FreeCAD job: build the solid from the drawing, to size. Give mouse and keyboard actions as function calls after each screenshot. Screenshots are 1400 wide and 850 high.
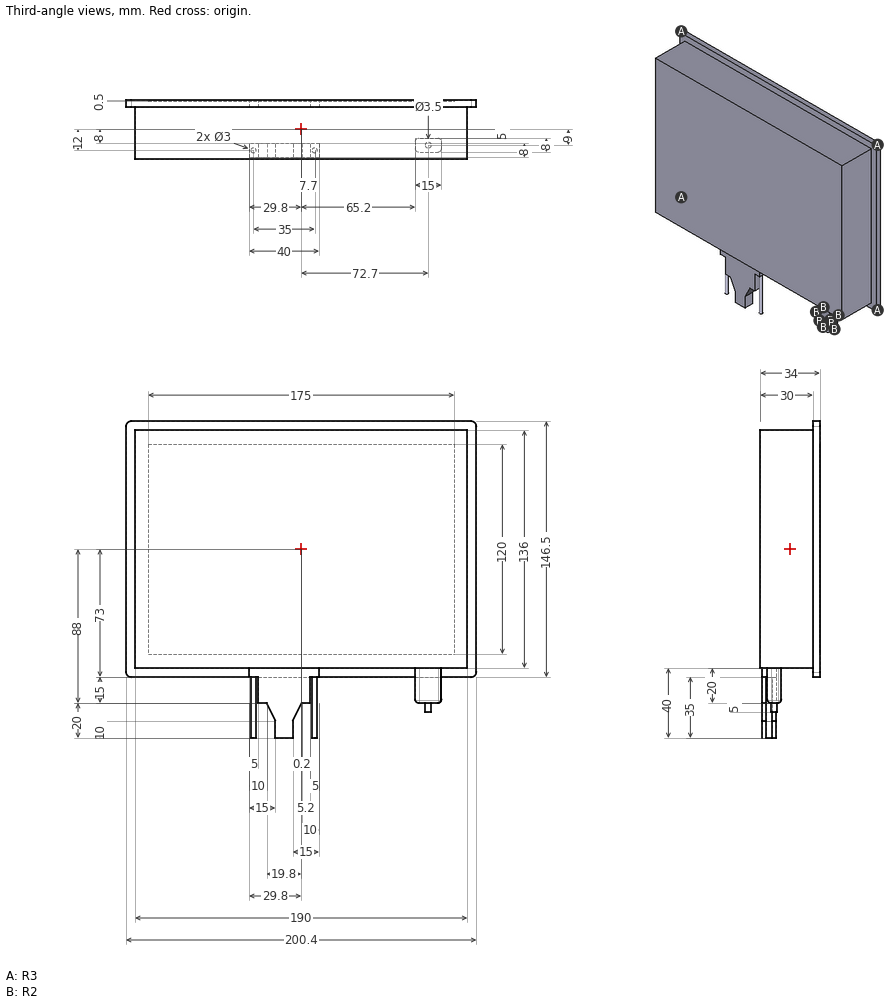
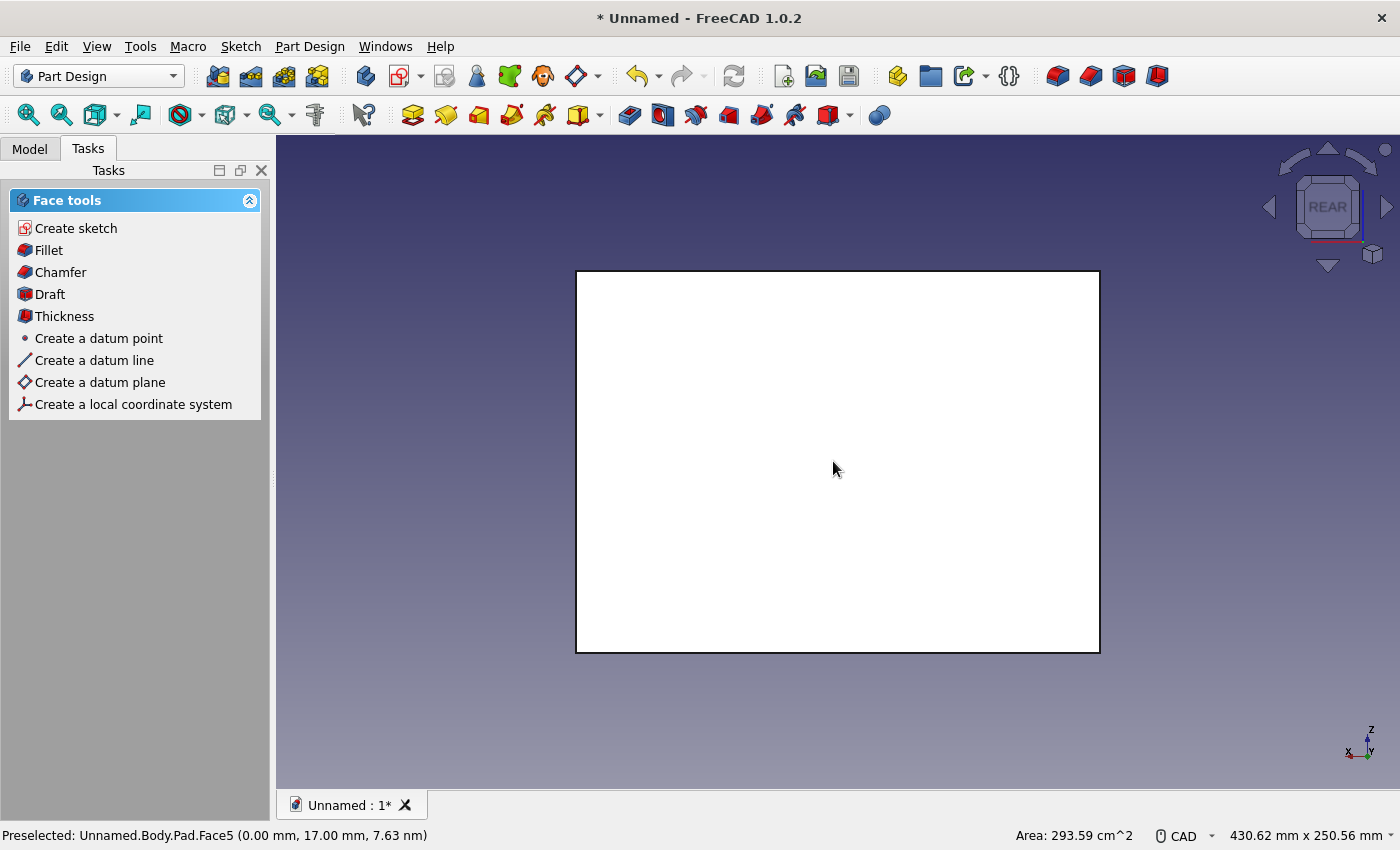
click(398, 76)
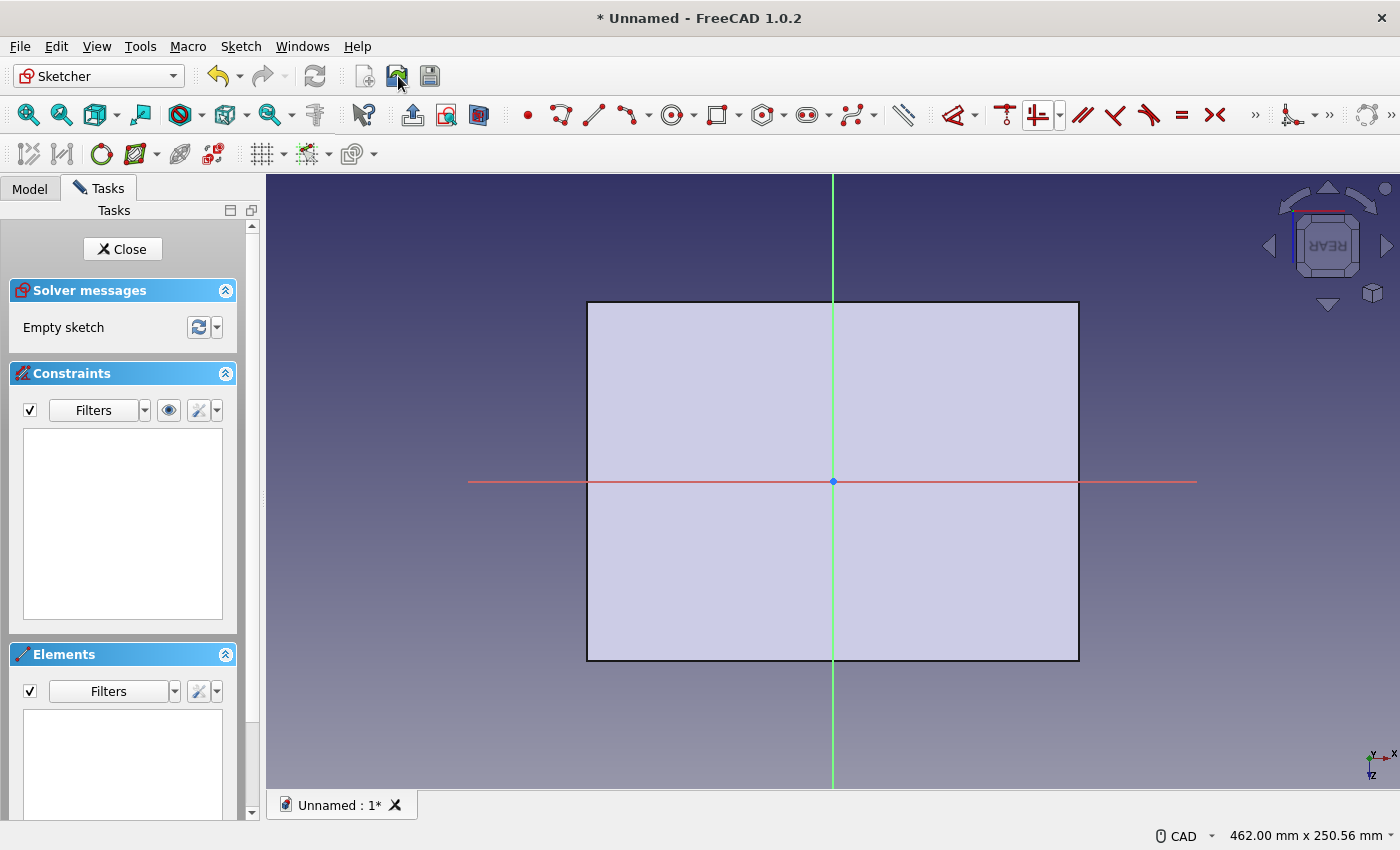
key(g)
key(v)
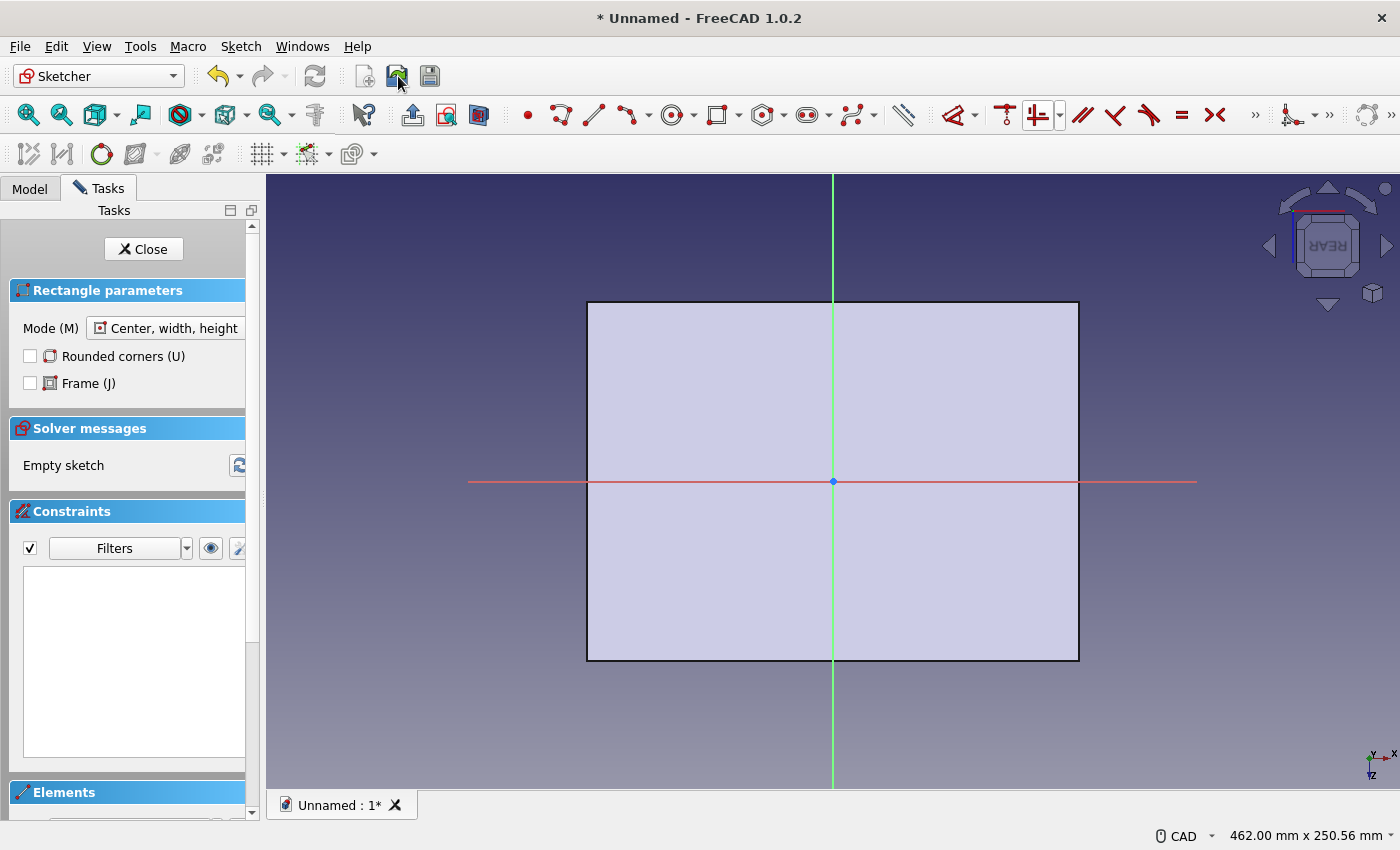
click(833, 481)
move(1048, 334)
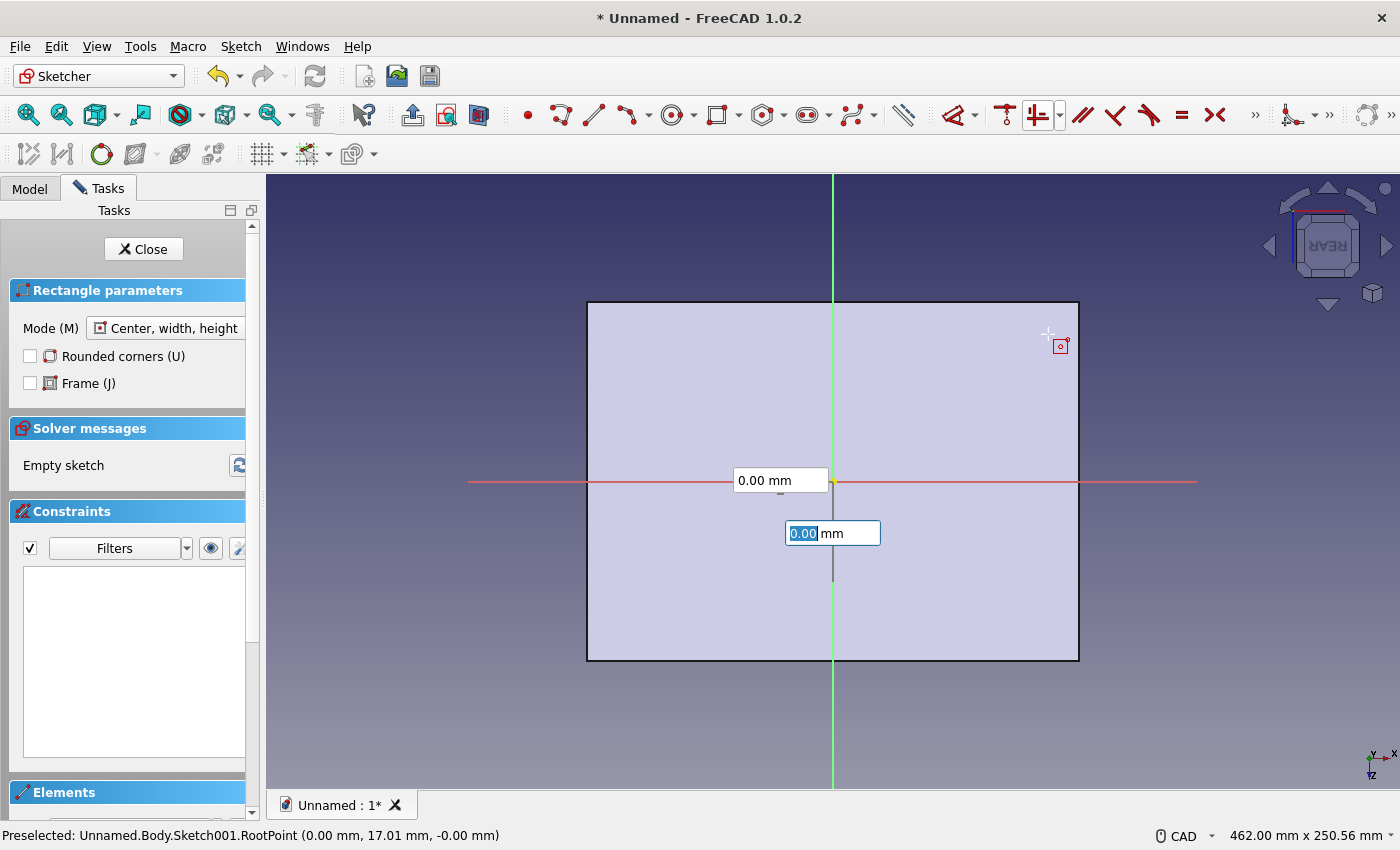
text(175)
key(Tab)
text(120)
key(Return)
key(Escape)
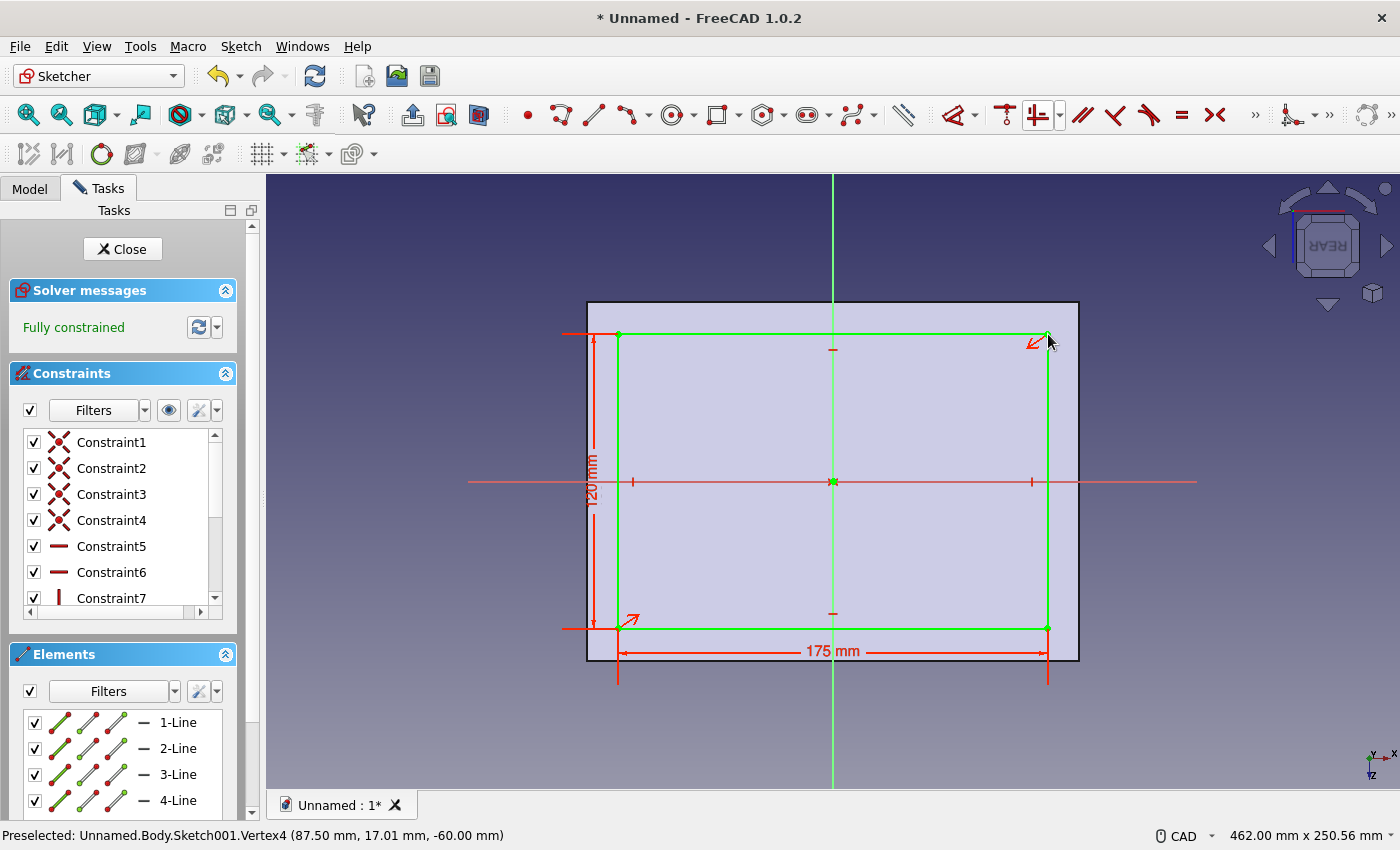
click(123, 249)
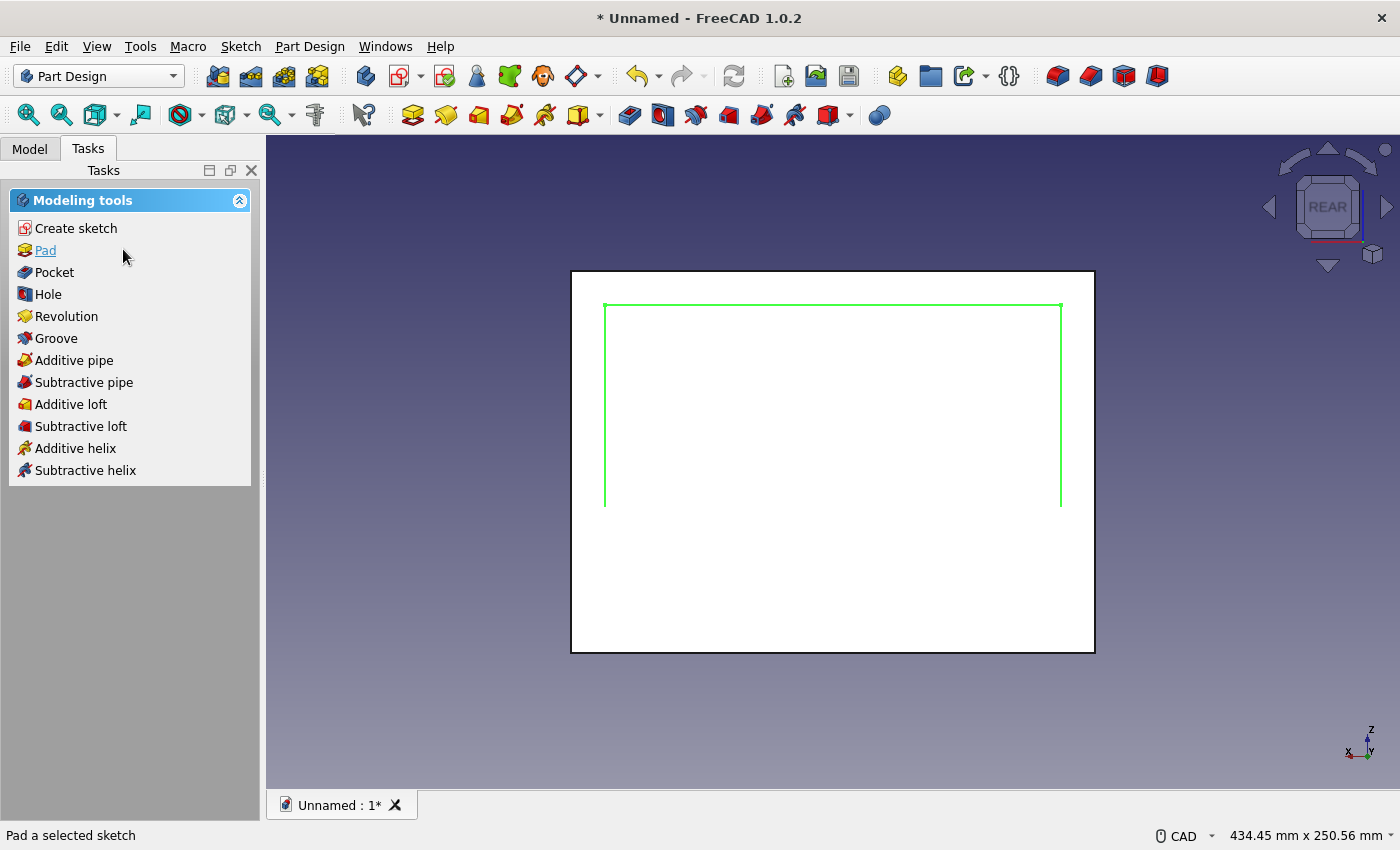
click(630, 116)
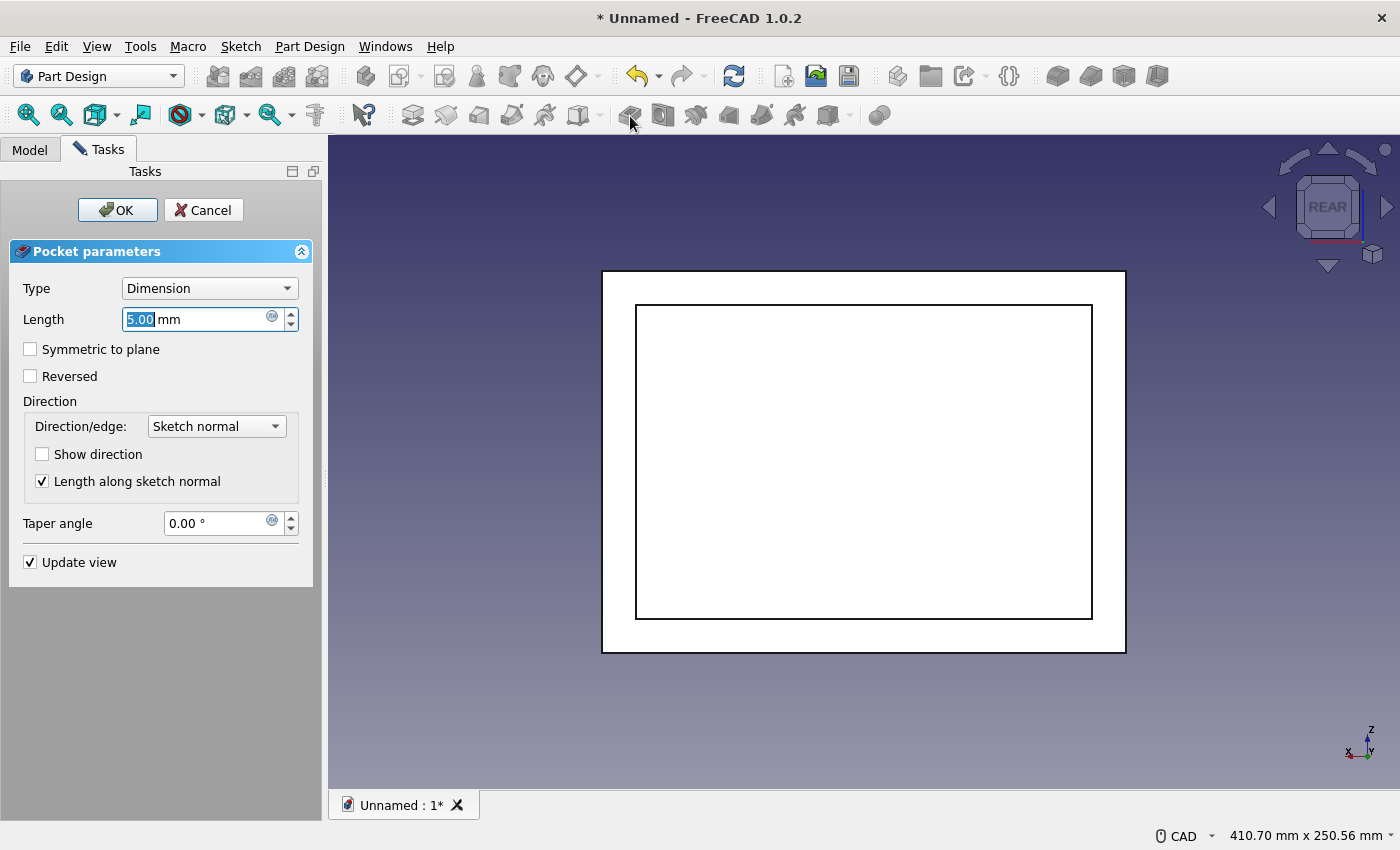
text(0.5)
key(Tab)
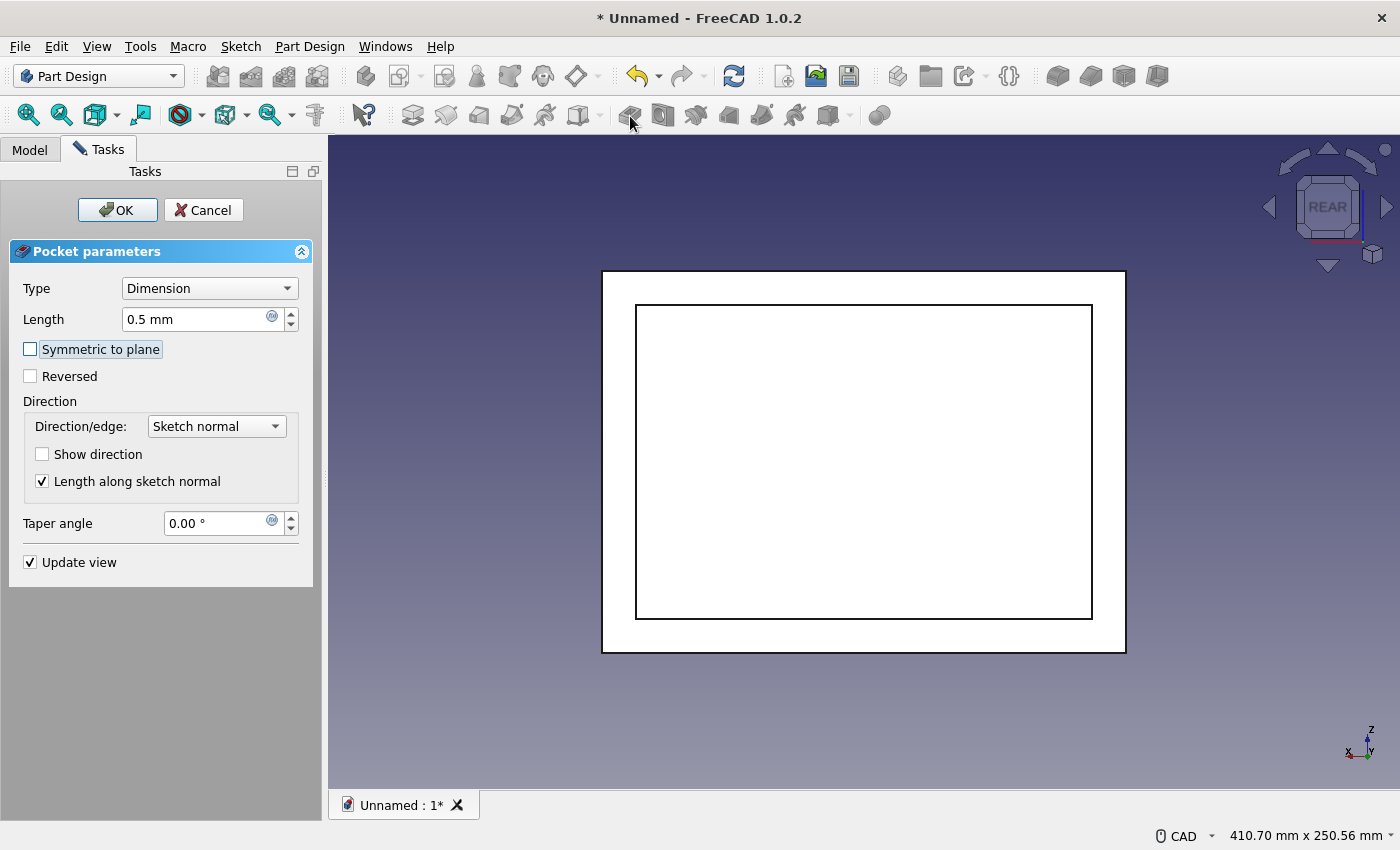
click(118, 210)